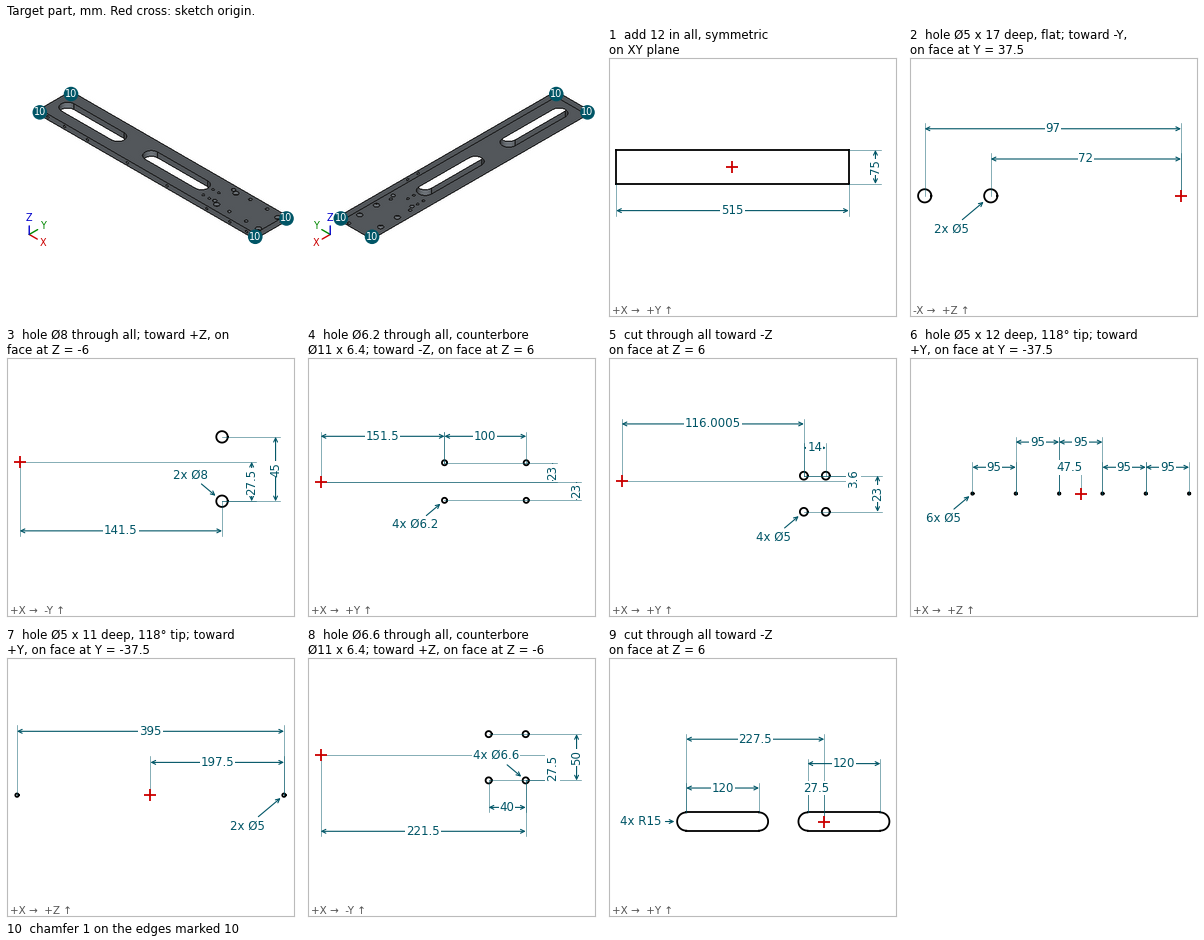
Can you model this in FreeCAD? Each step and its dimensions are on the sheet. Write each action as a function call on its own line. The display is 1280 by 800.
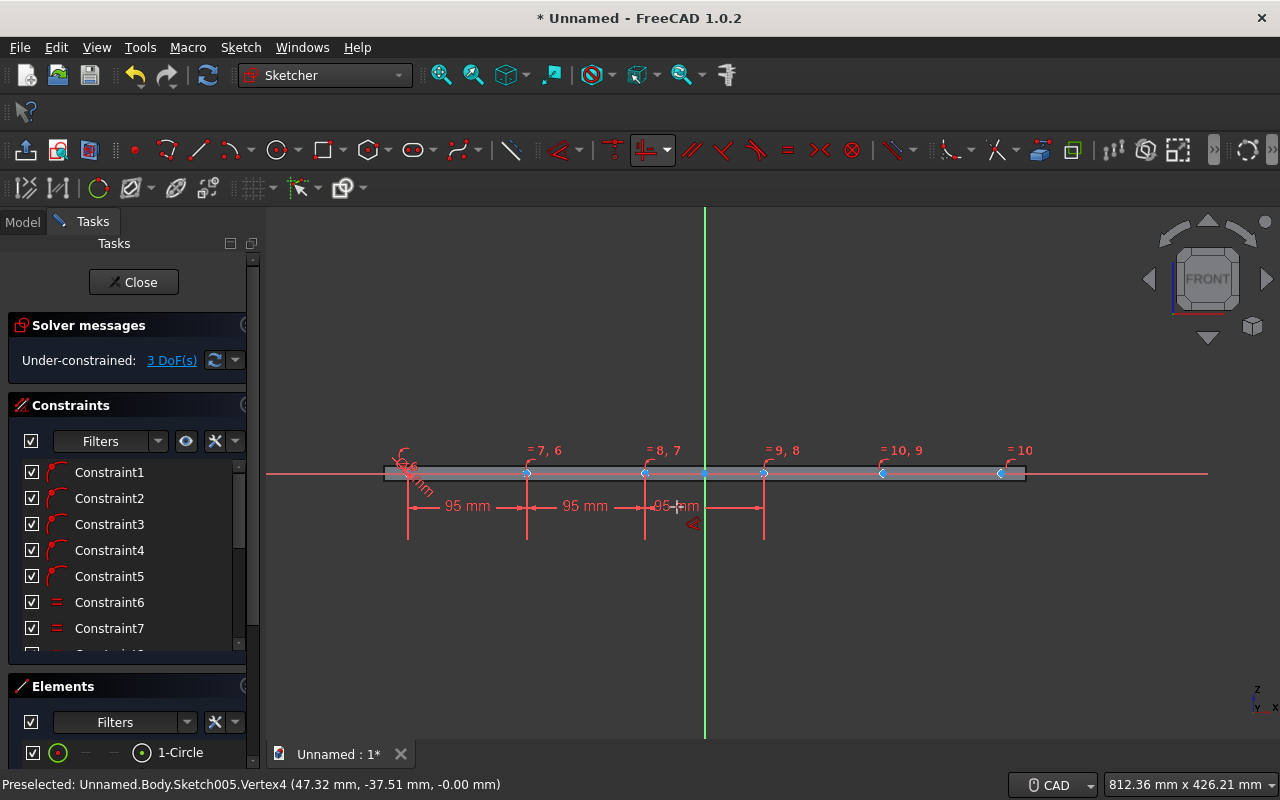
click(764, 473)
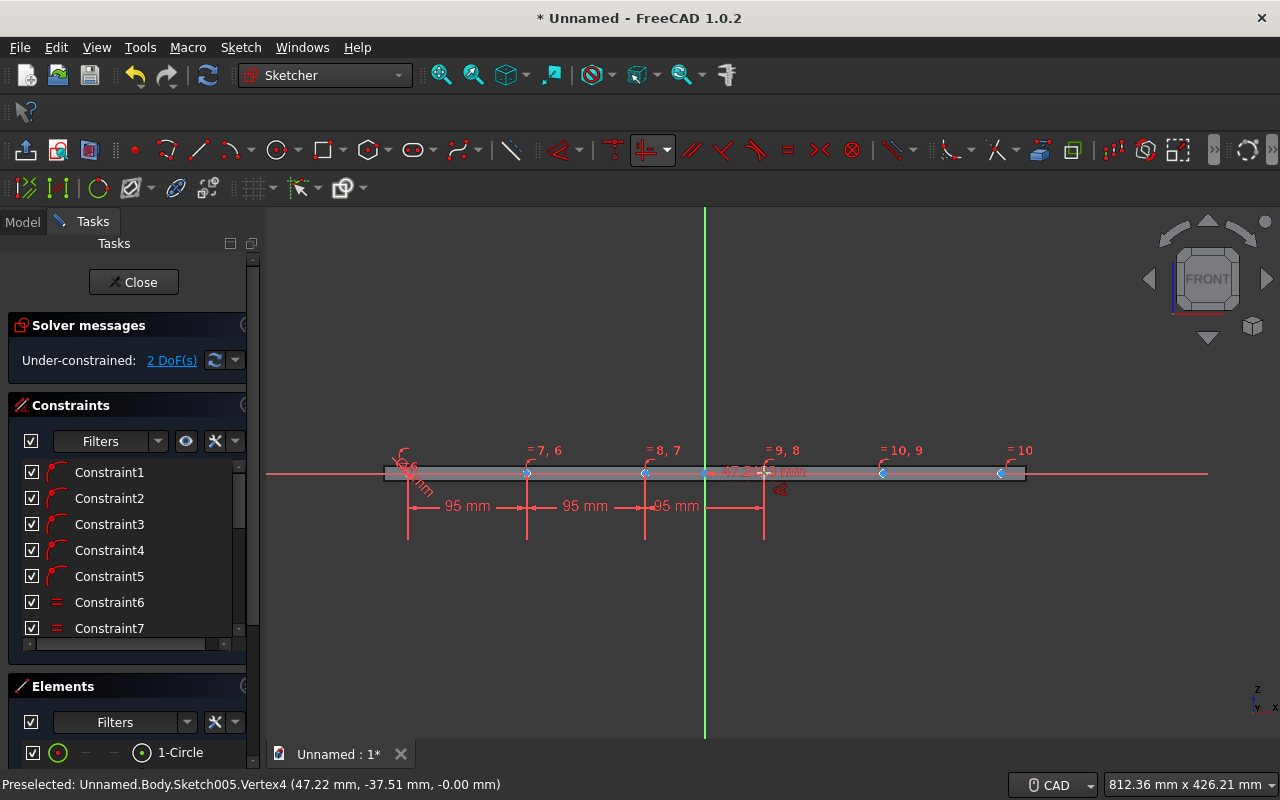
click(883, 473)
click(823, 507)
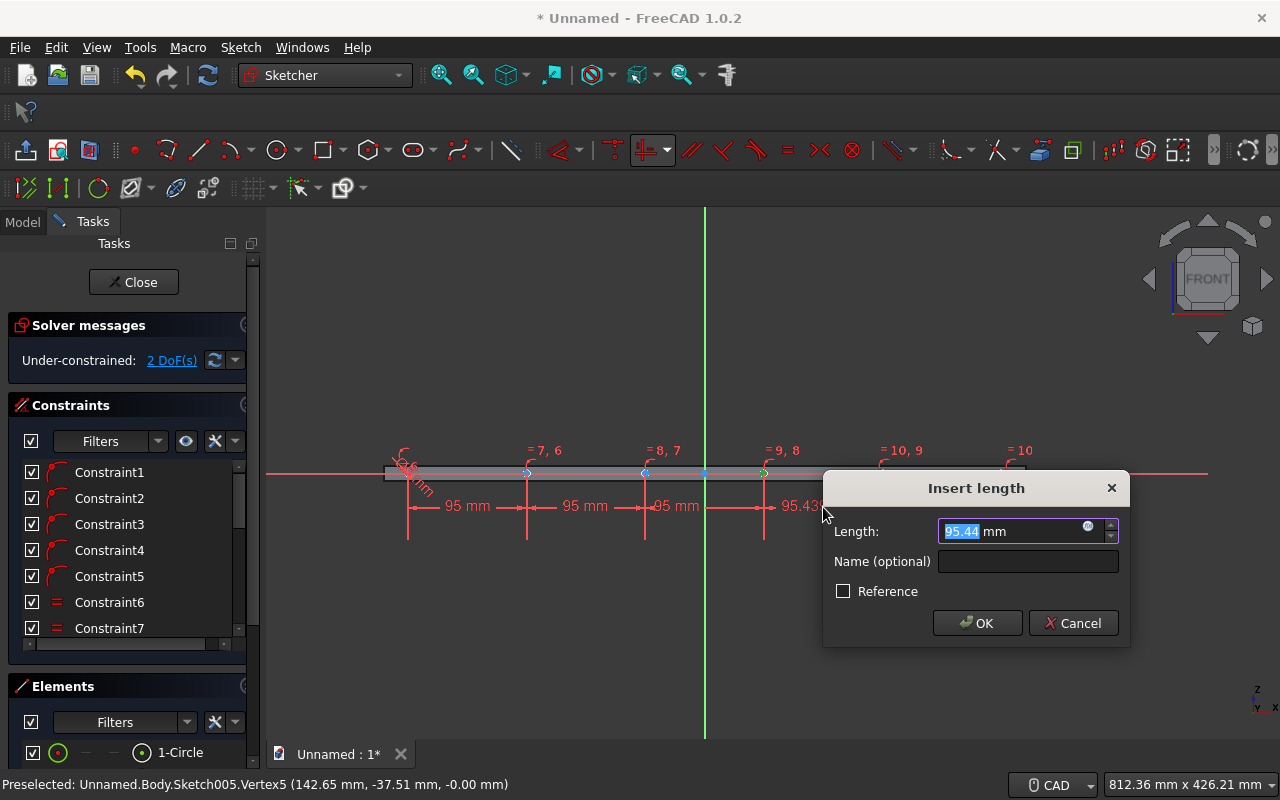
text(95)
key(Return)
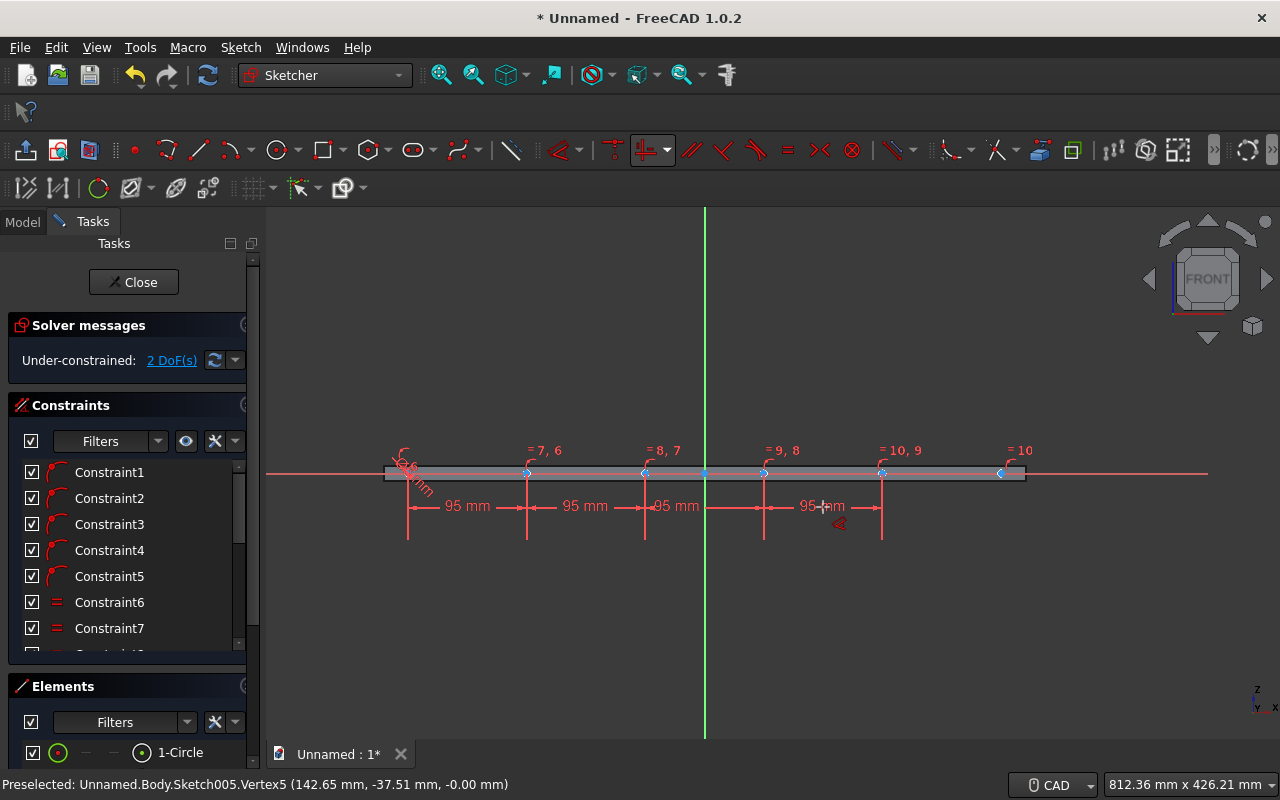
click(882, 473)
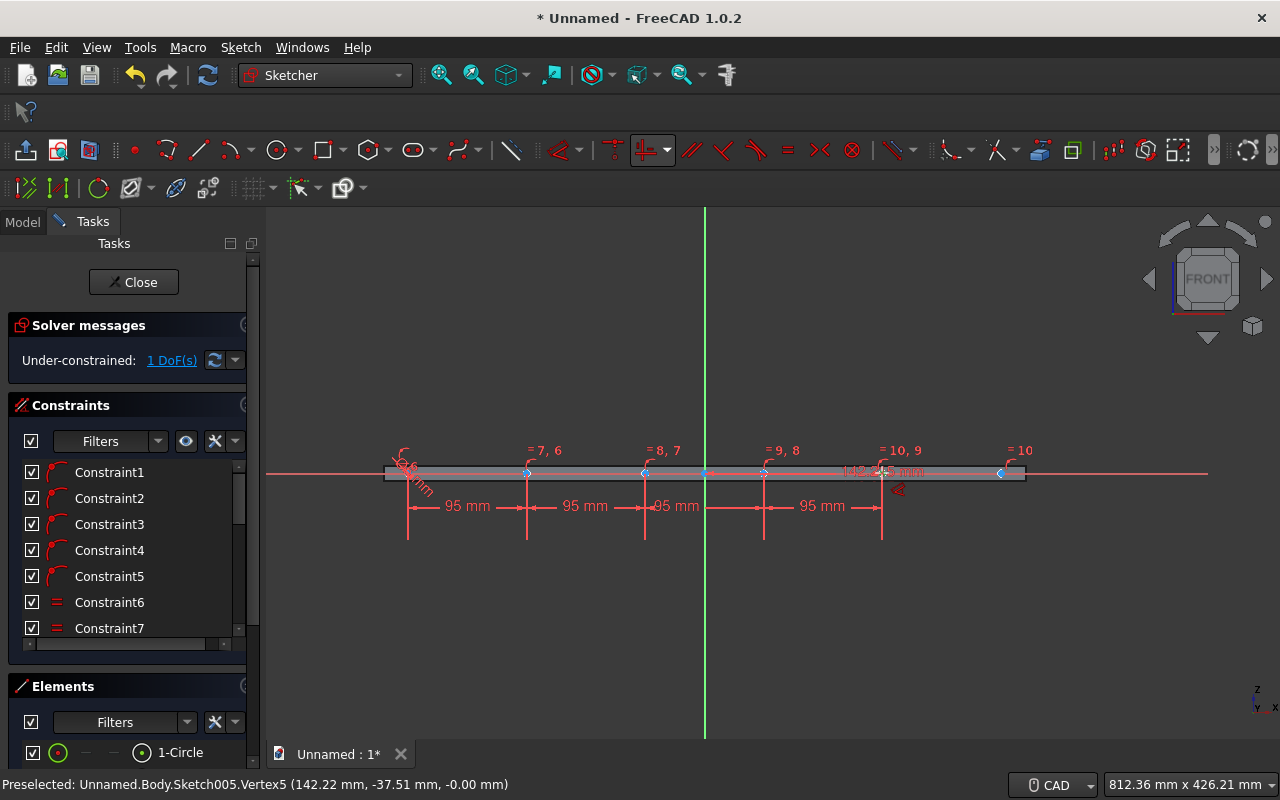
click(1001, 473)
click(942, 507)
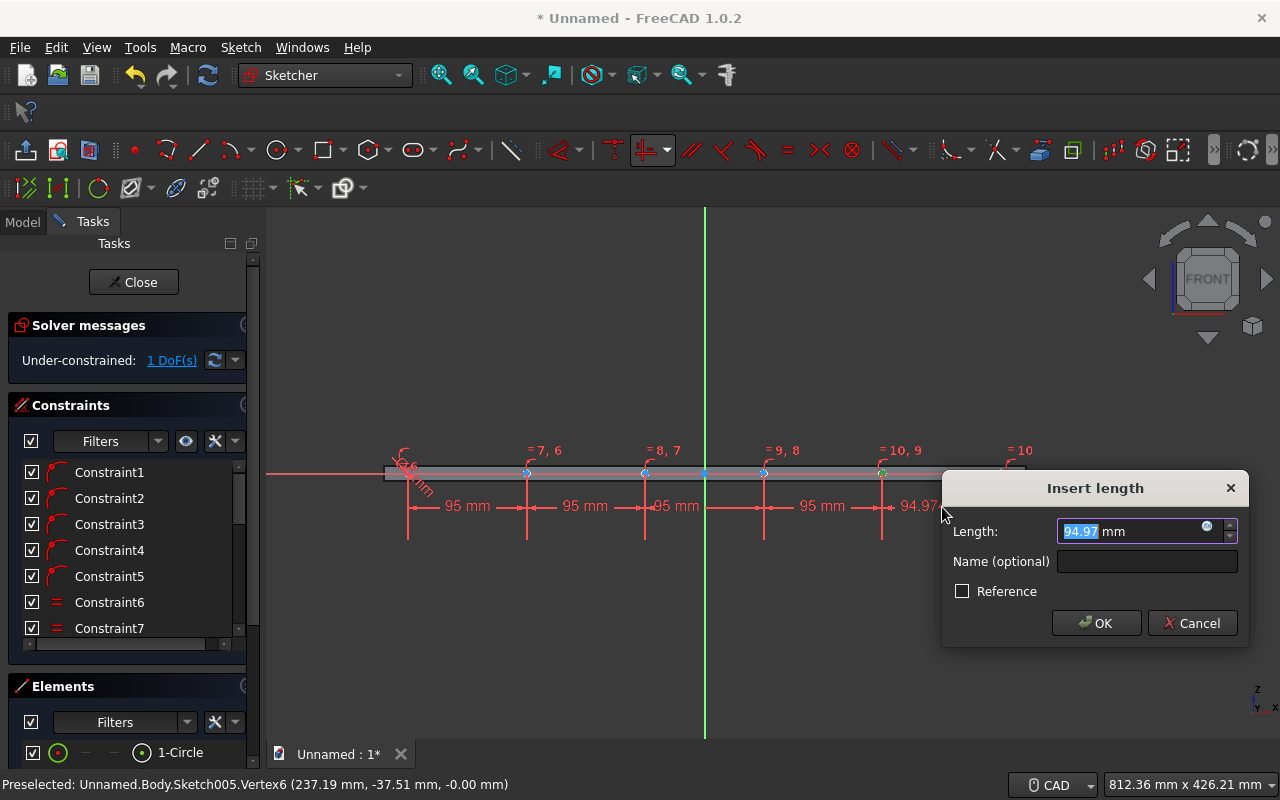
text(95)
key(Return)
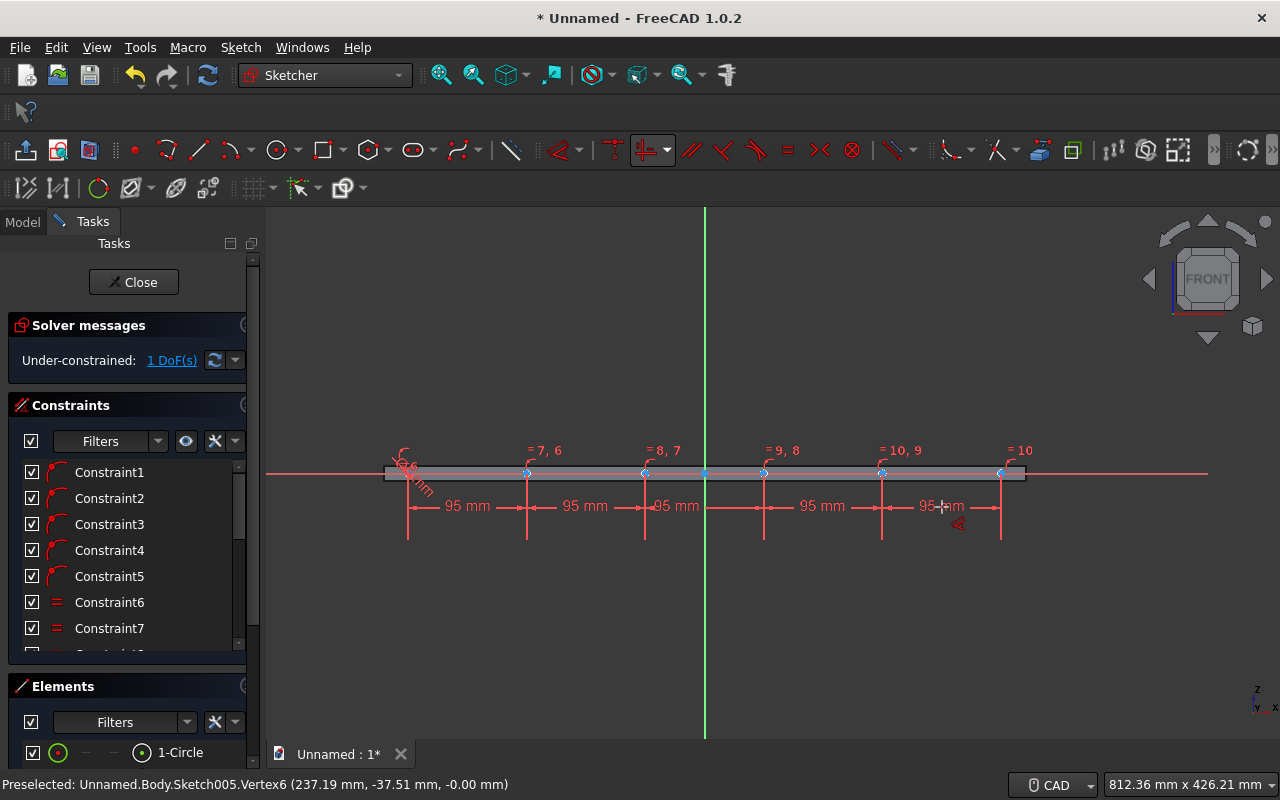
click(645, 473)
click(675, 439)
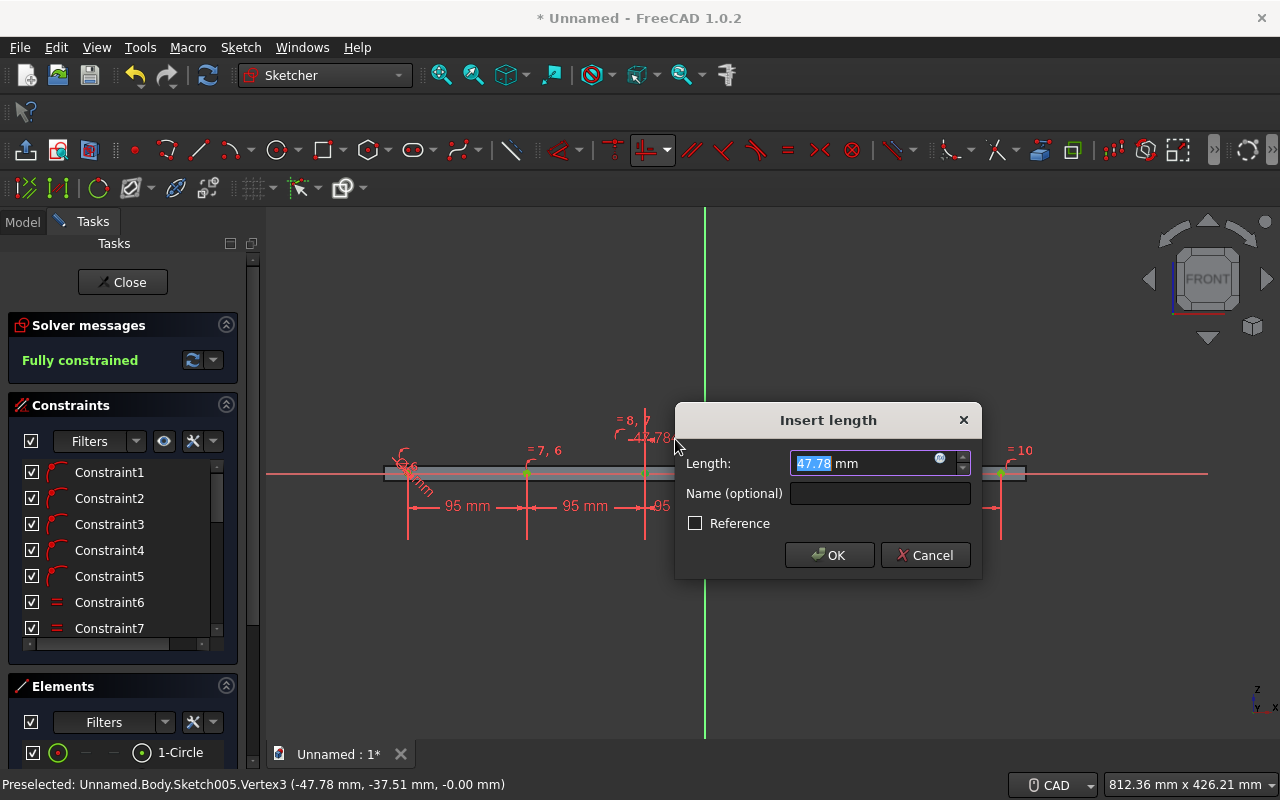
text(47.5)
key(Return)
key(Escape)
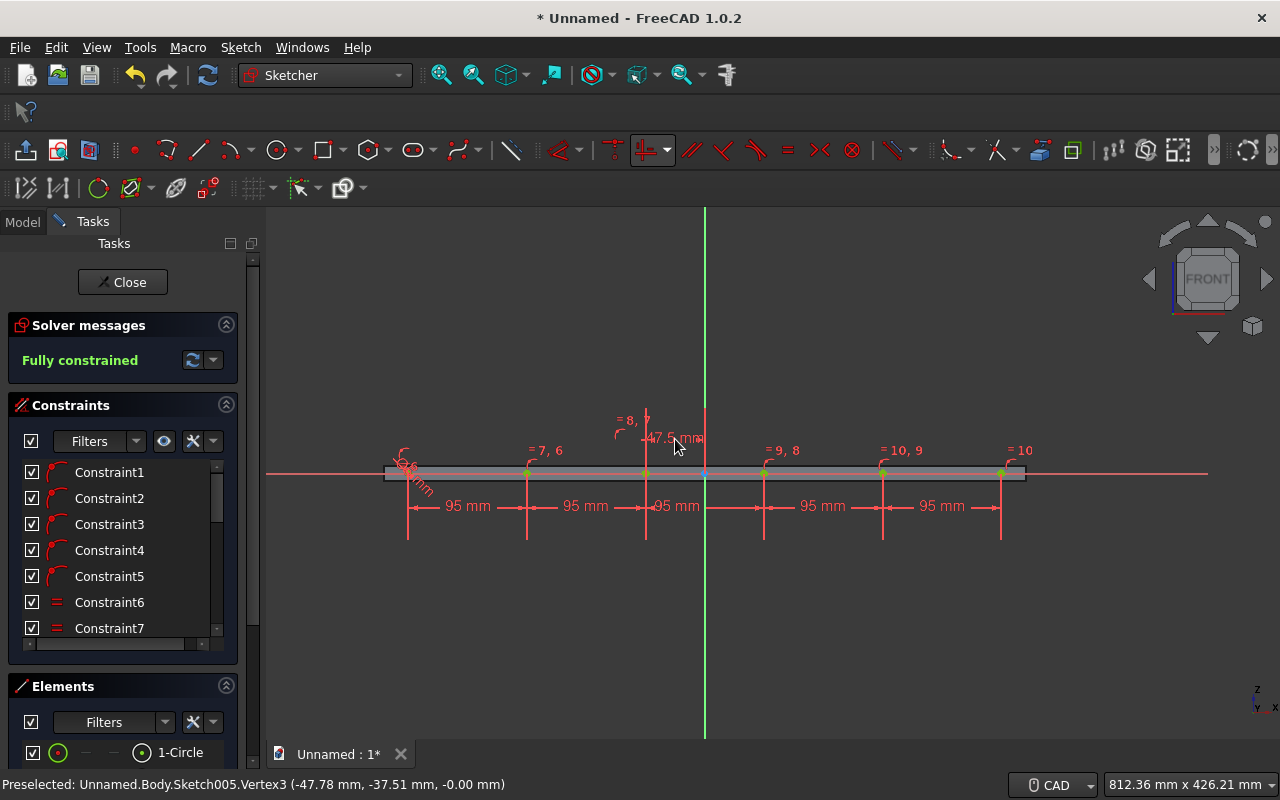
click(123, 282)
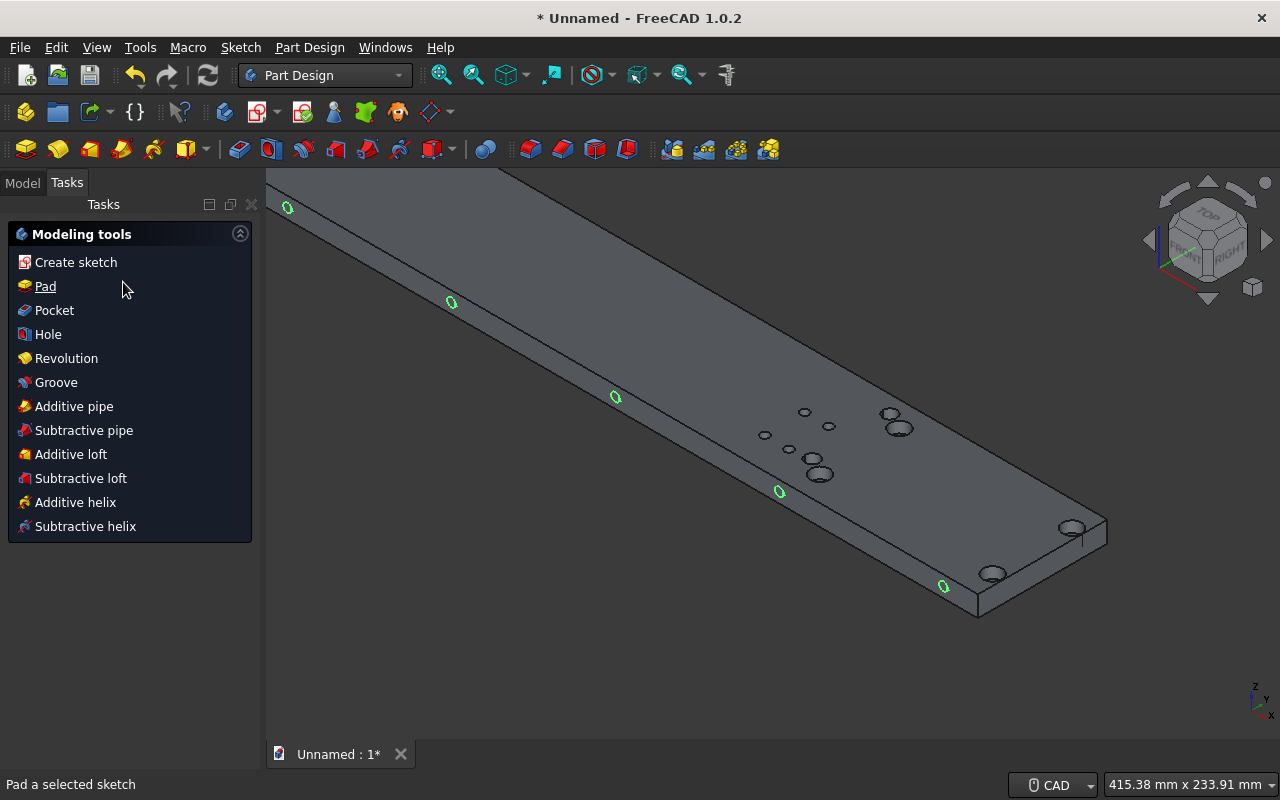
click(272, 150)